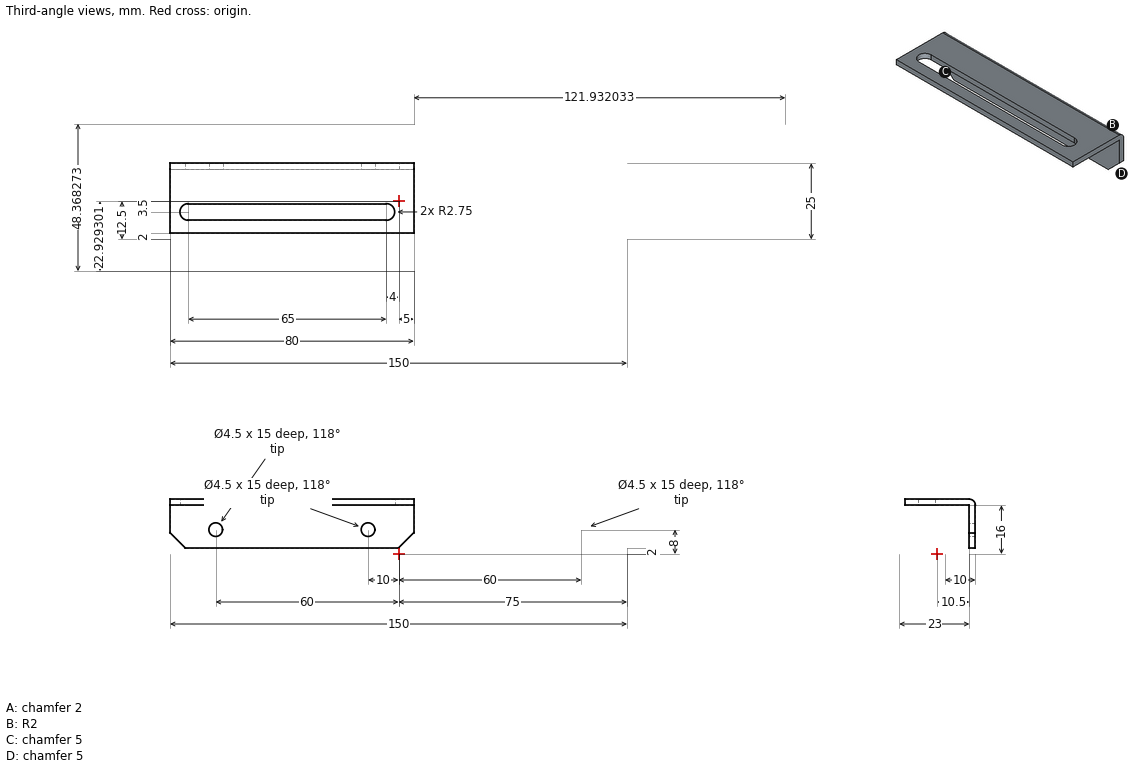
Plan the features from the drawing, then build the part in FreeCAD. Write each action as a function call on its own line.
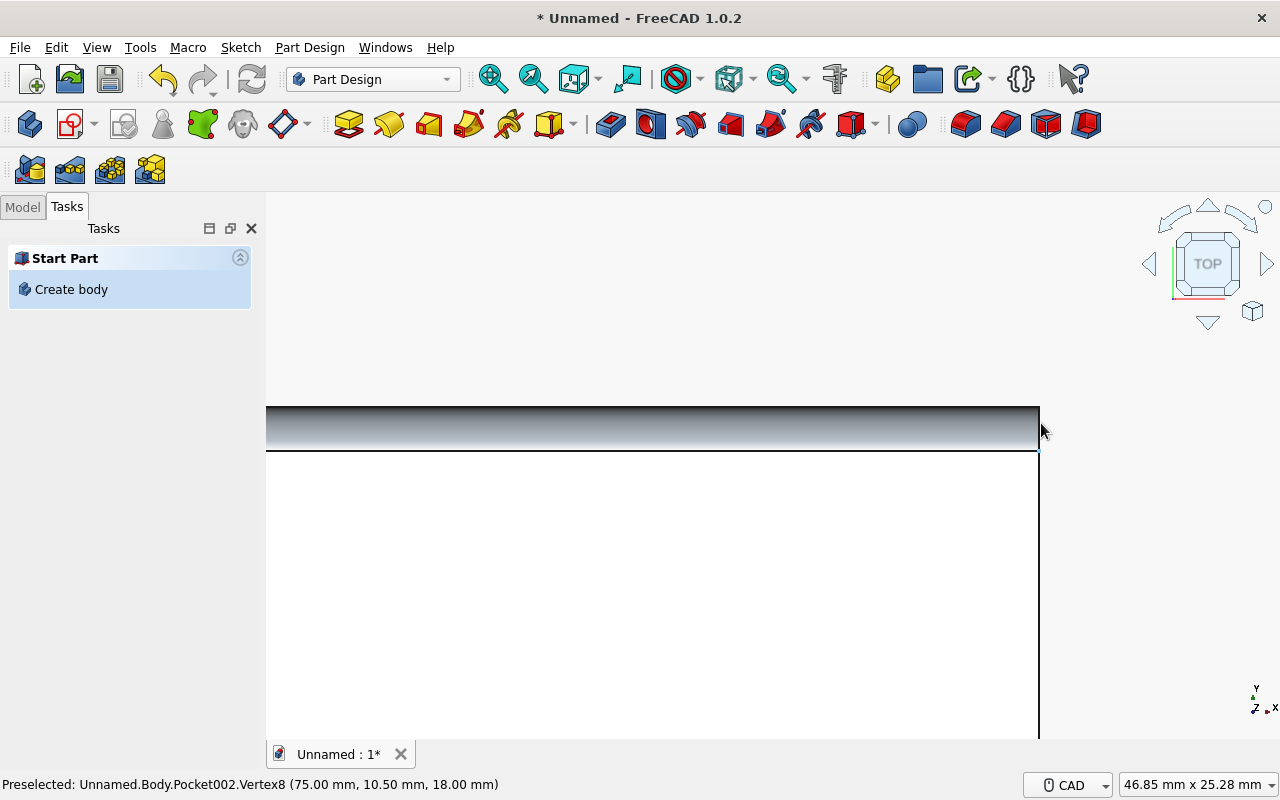
click(494, 80)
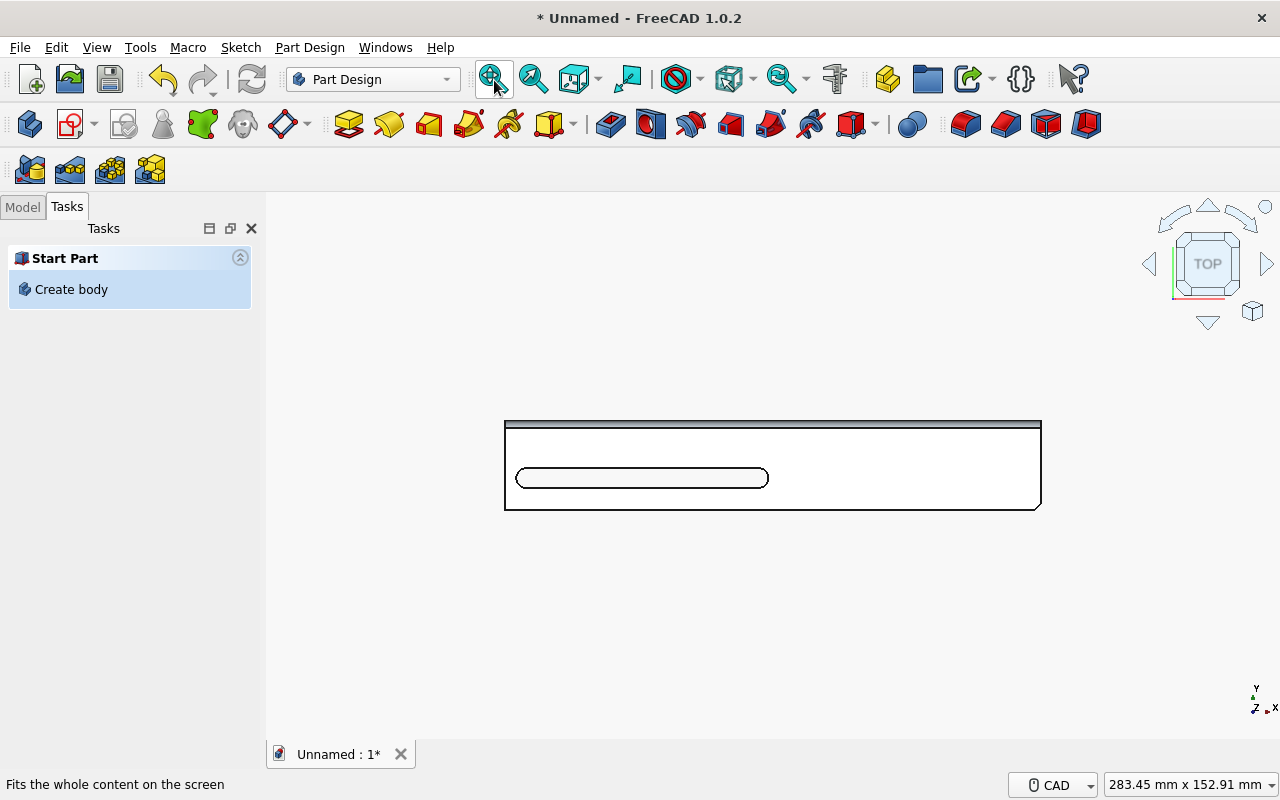
key(1)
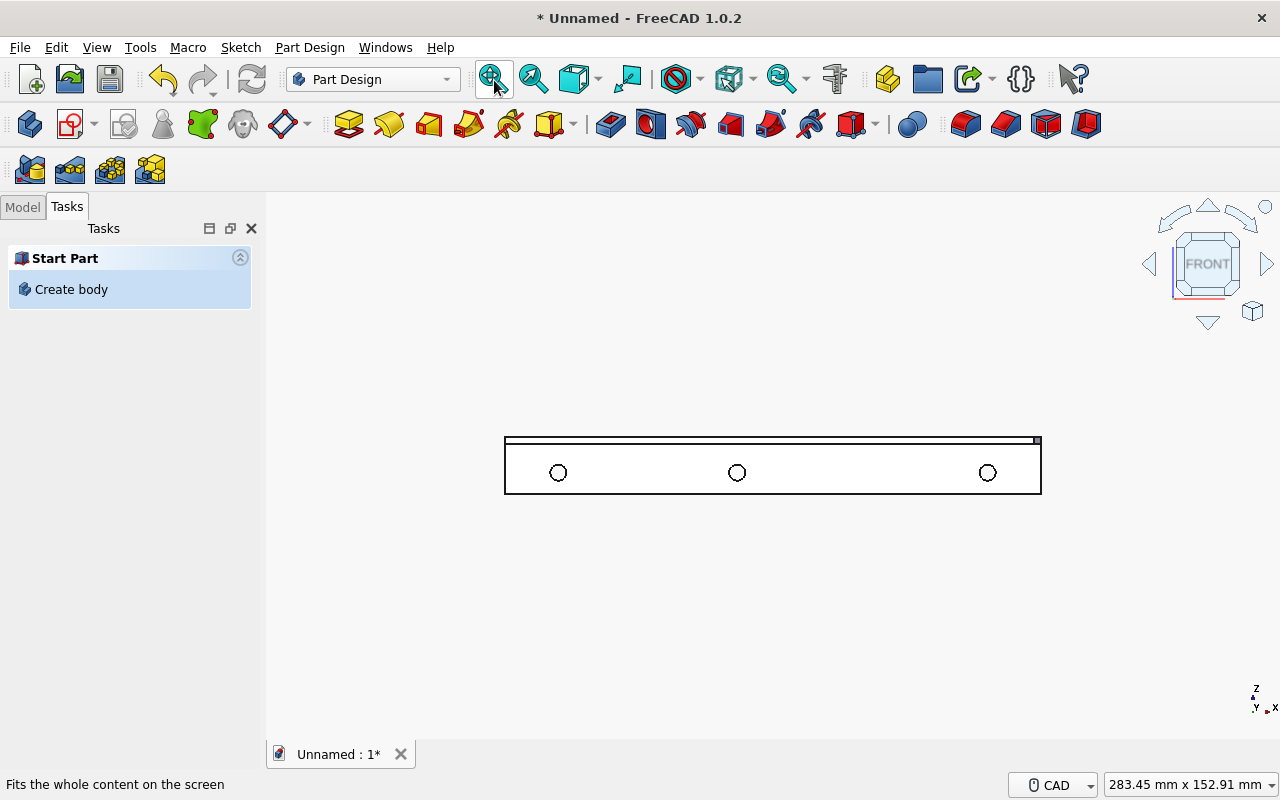
scroll(1041, 493, up, 9)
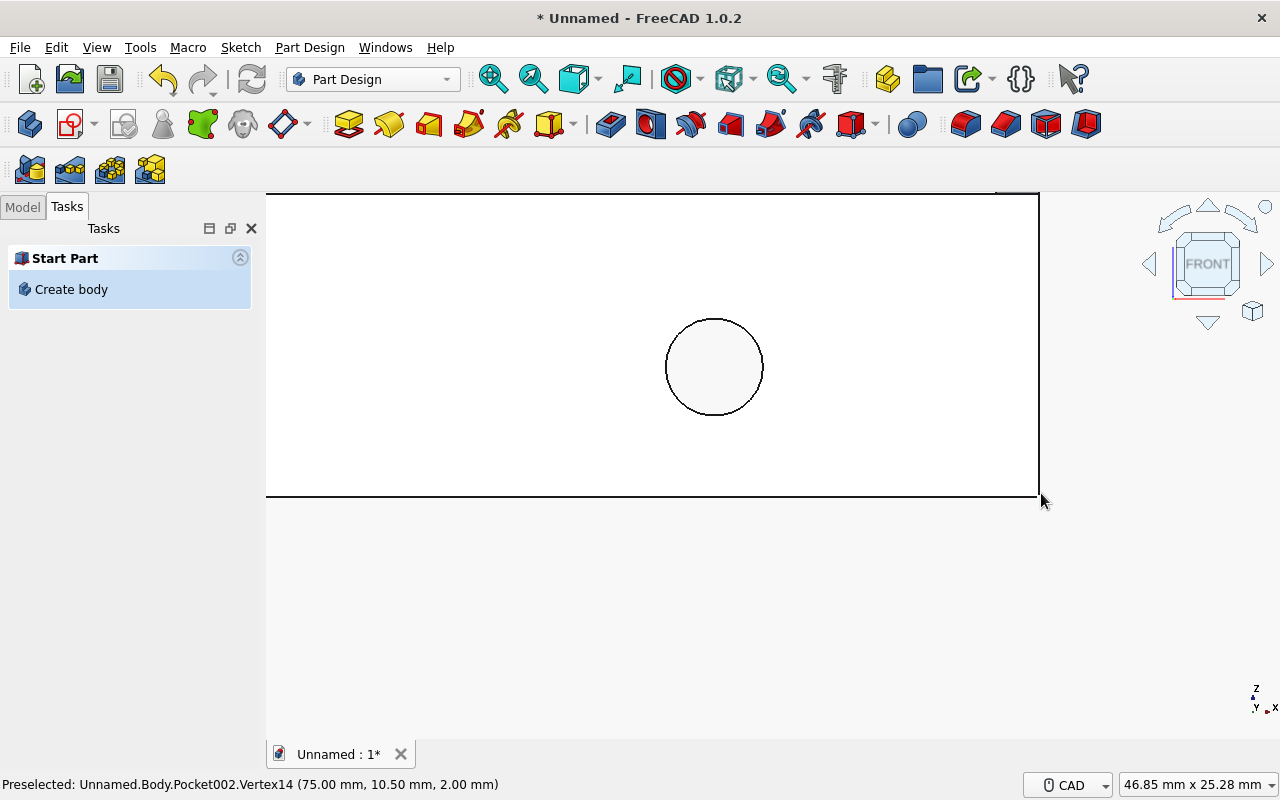
click(494, 80)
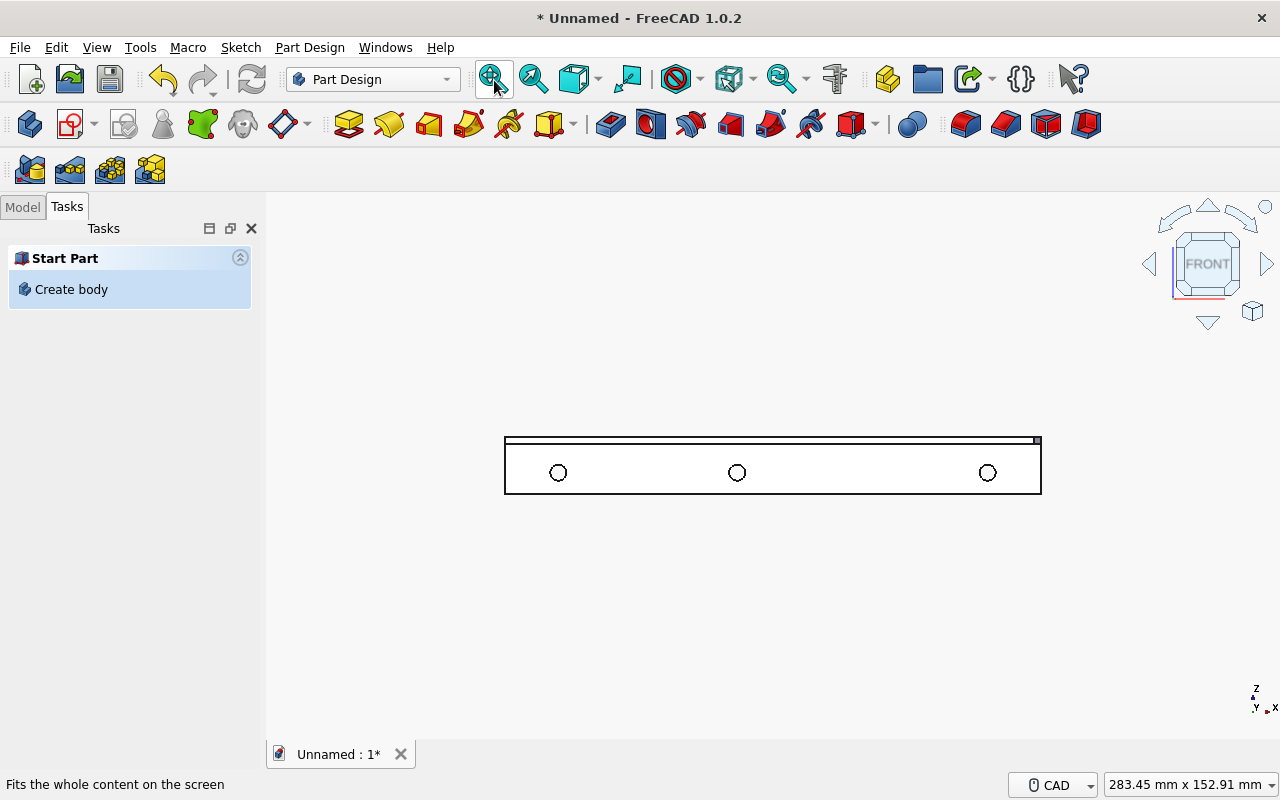
key(3)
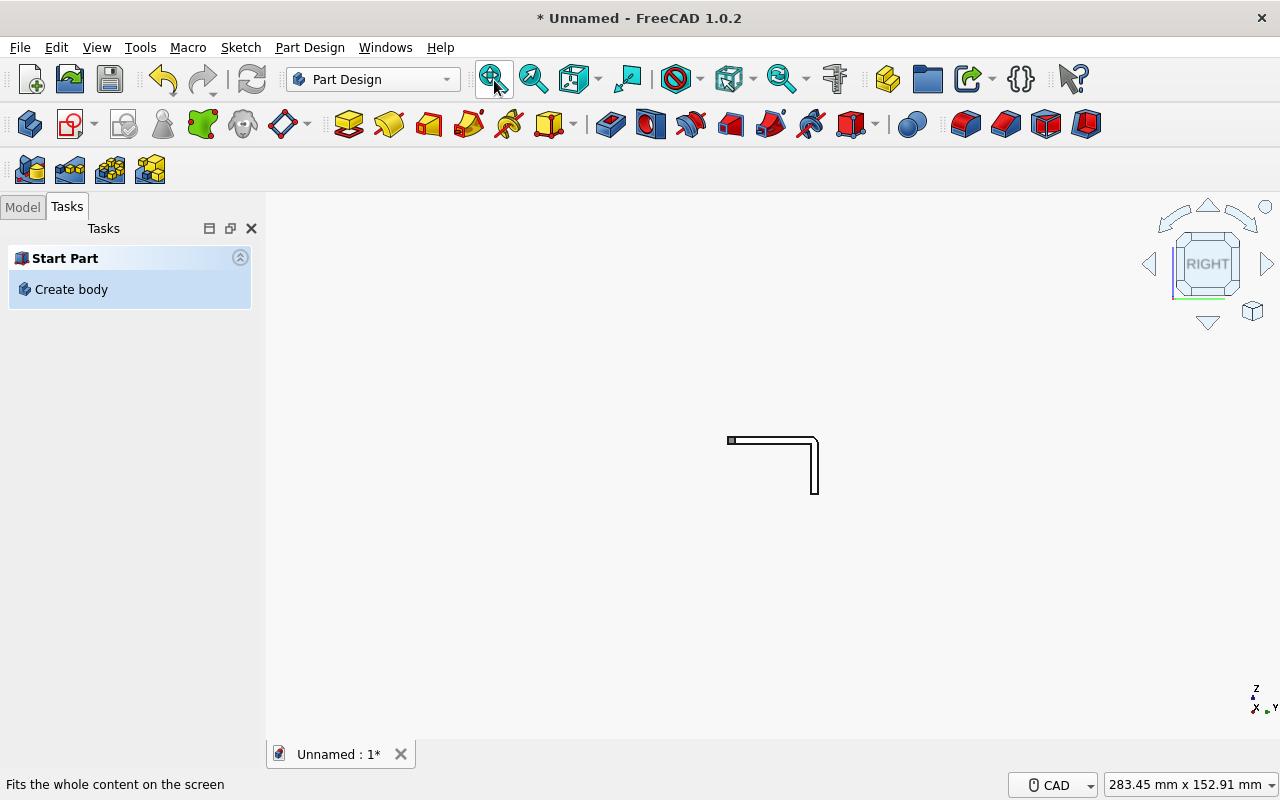
click(494, 80)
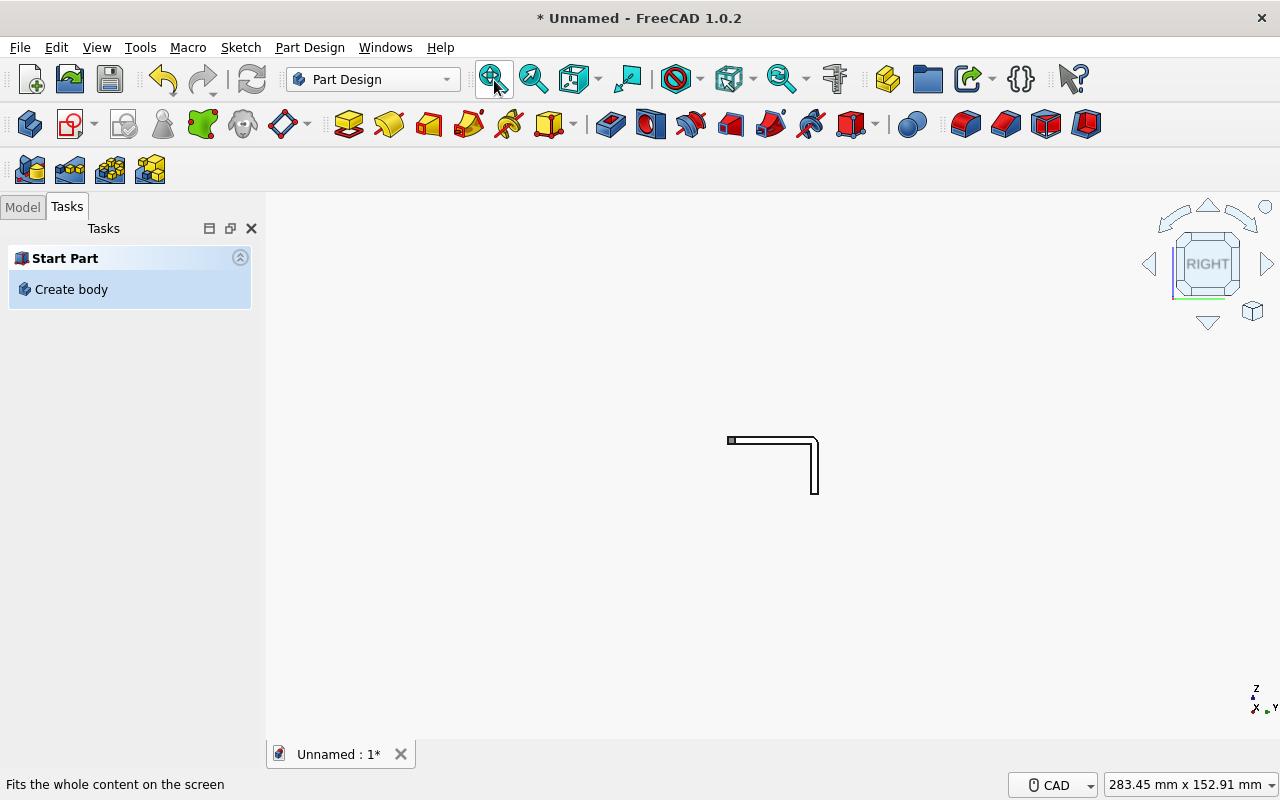
scroll(814, 493, up, 9)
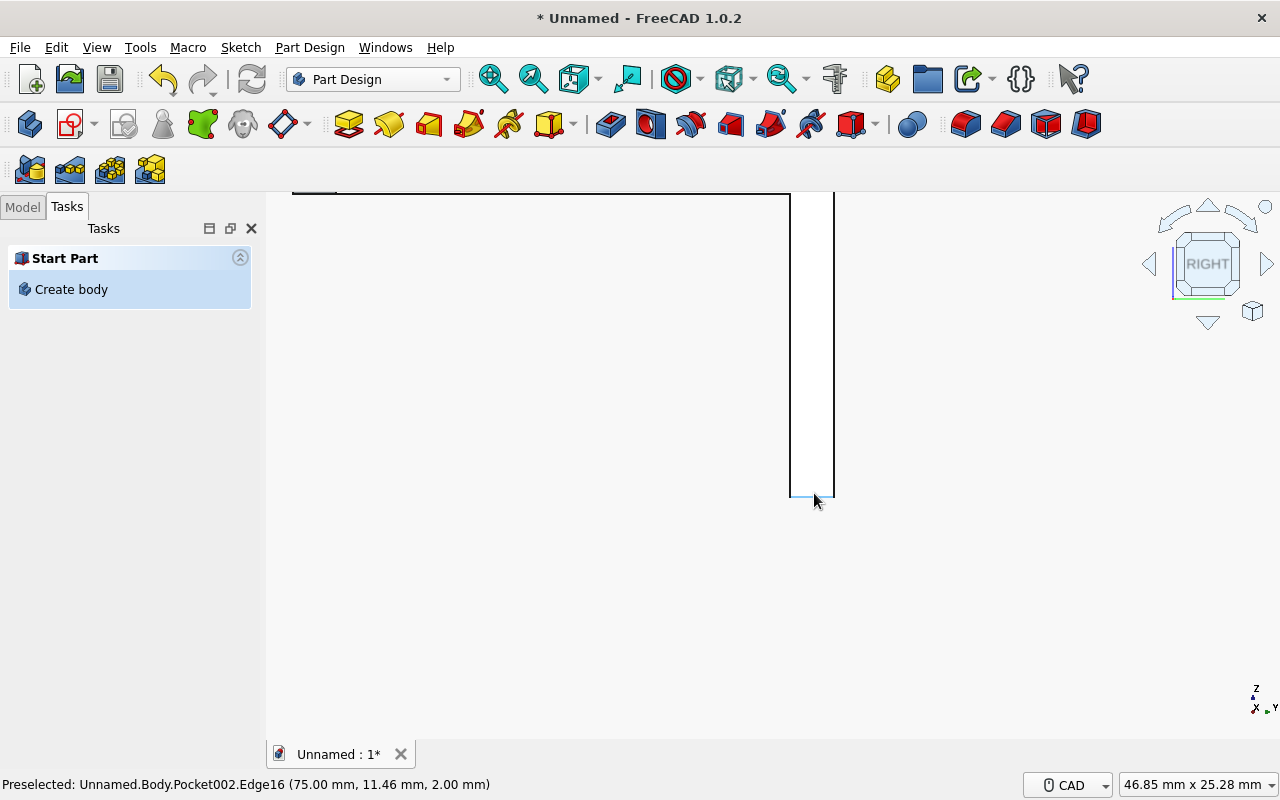
click(812, 496)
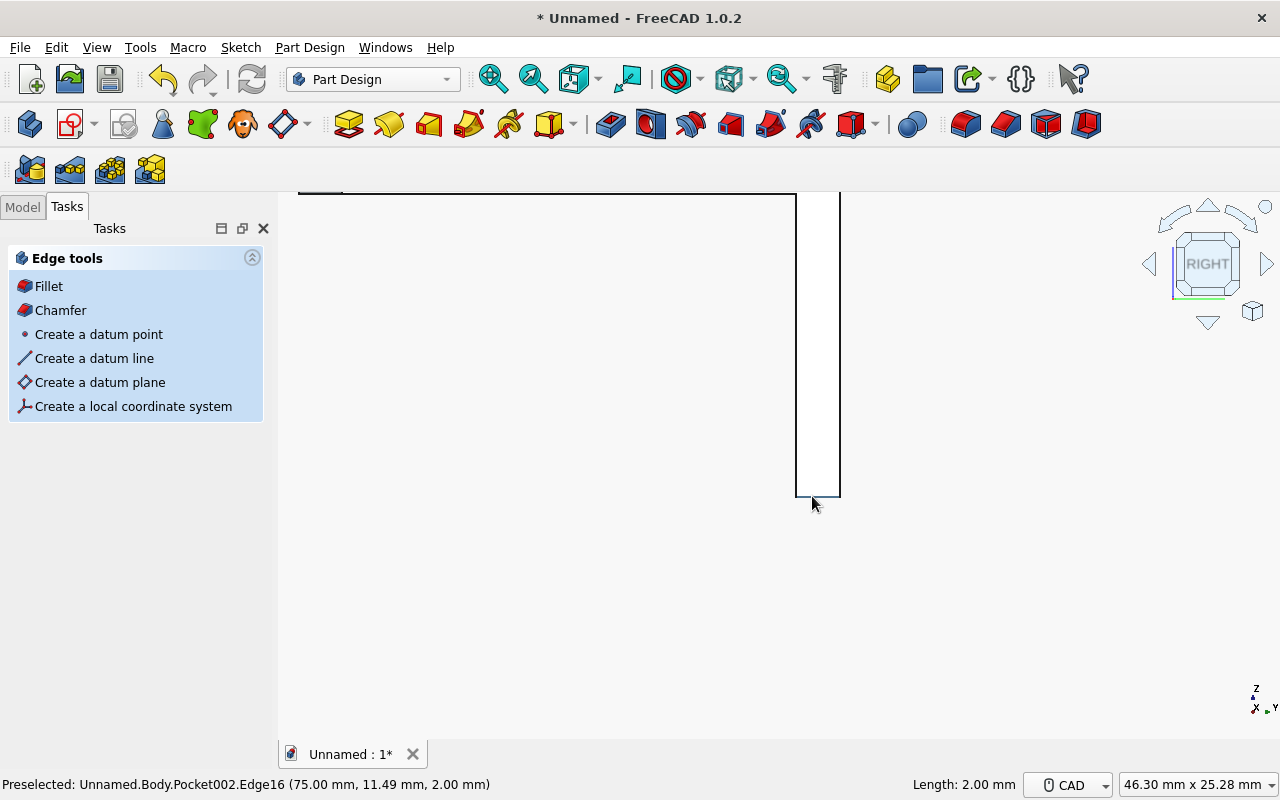
click(494, 80)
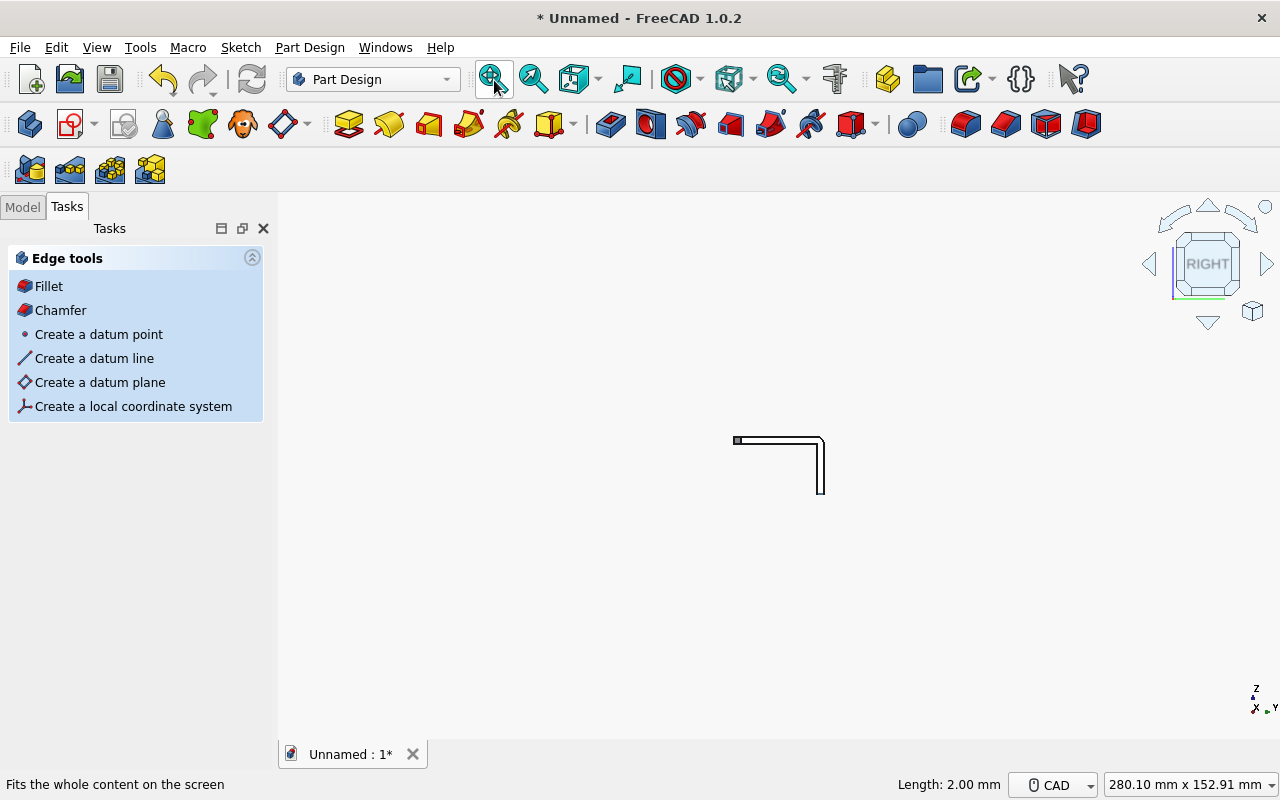
key(5)